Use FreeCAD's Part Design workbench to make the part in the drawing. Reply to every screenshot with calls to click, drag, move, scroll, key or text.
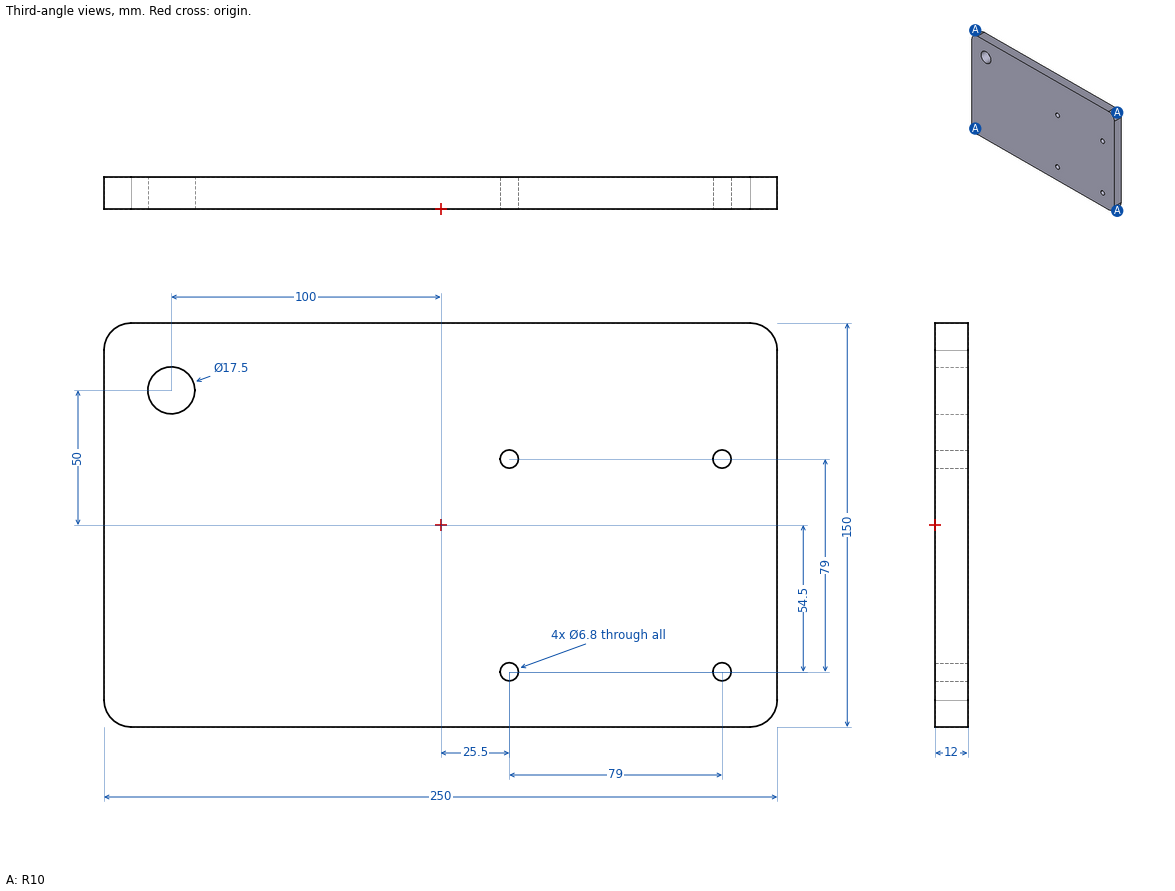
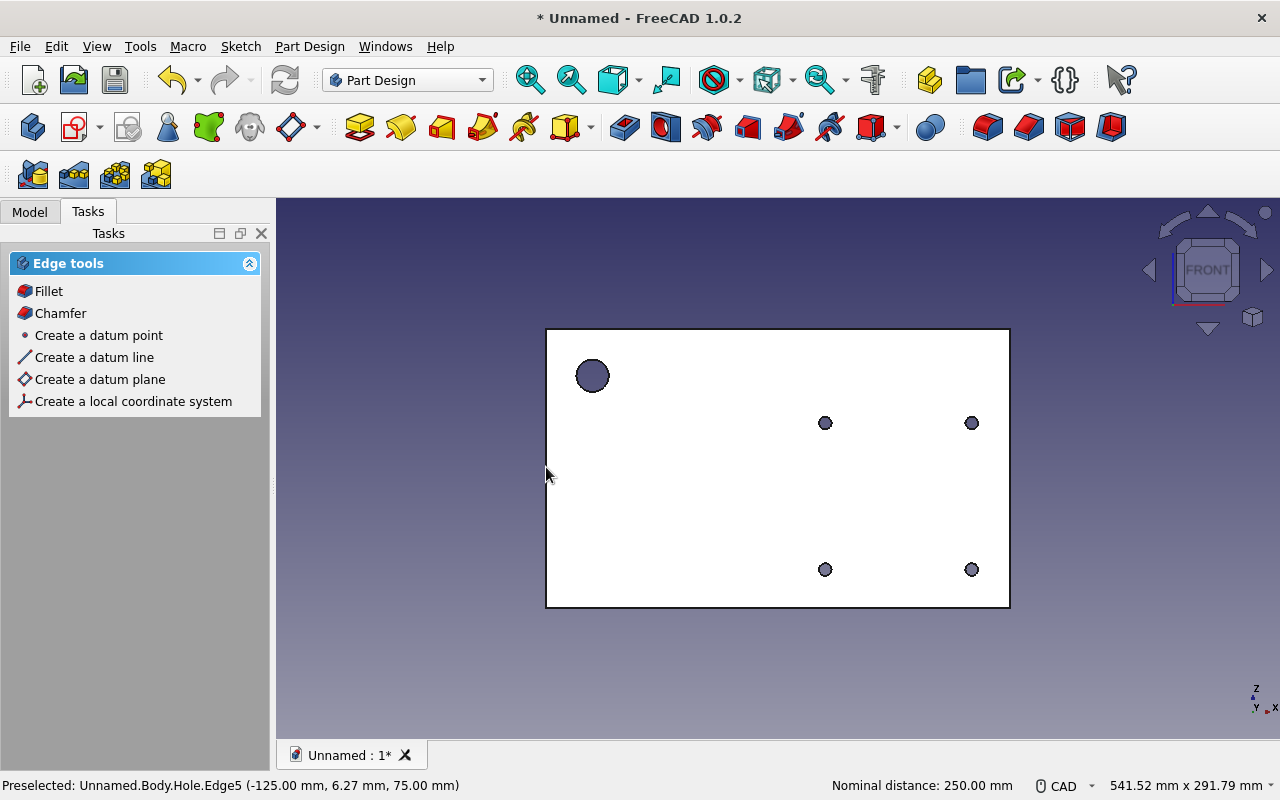
key(3)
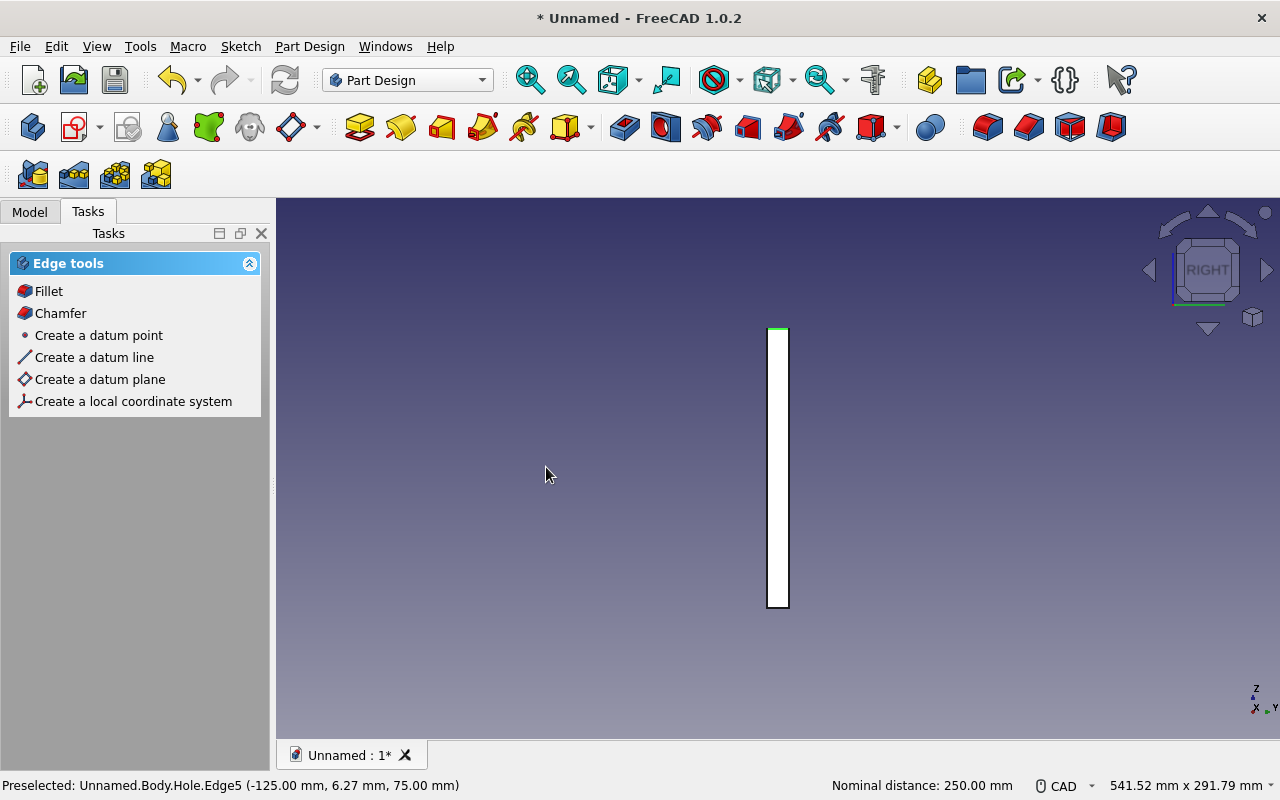
click(778, 607, ctrl)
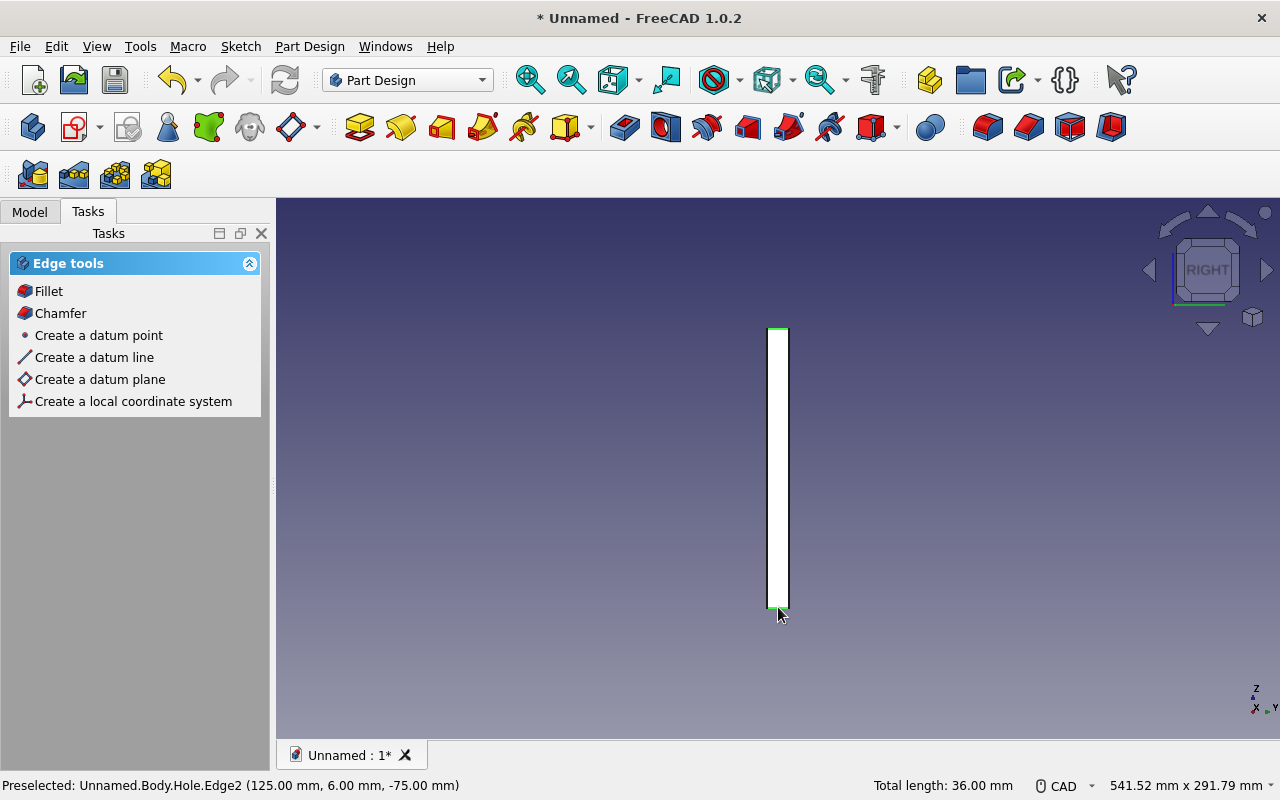
key(5)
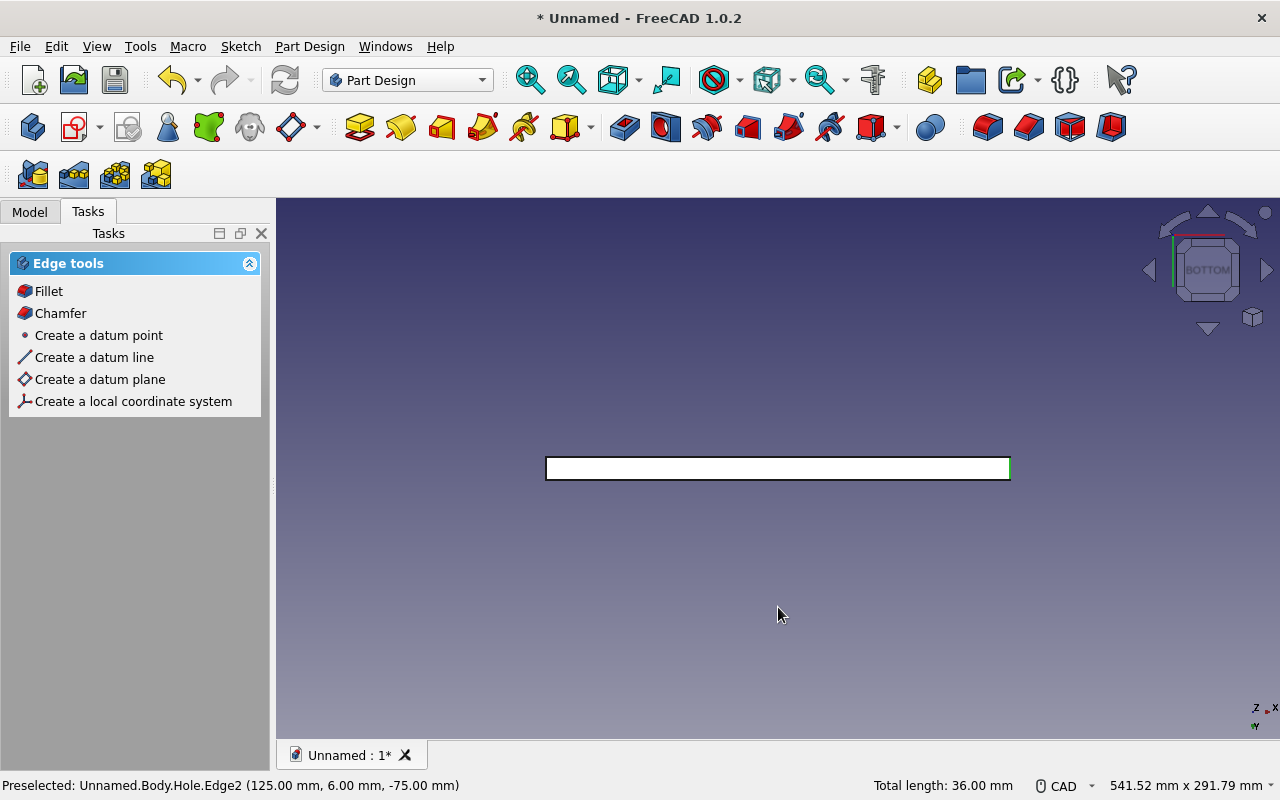
click(546, 468, ctrl)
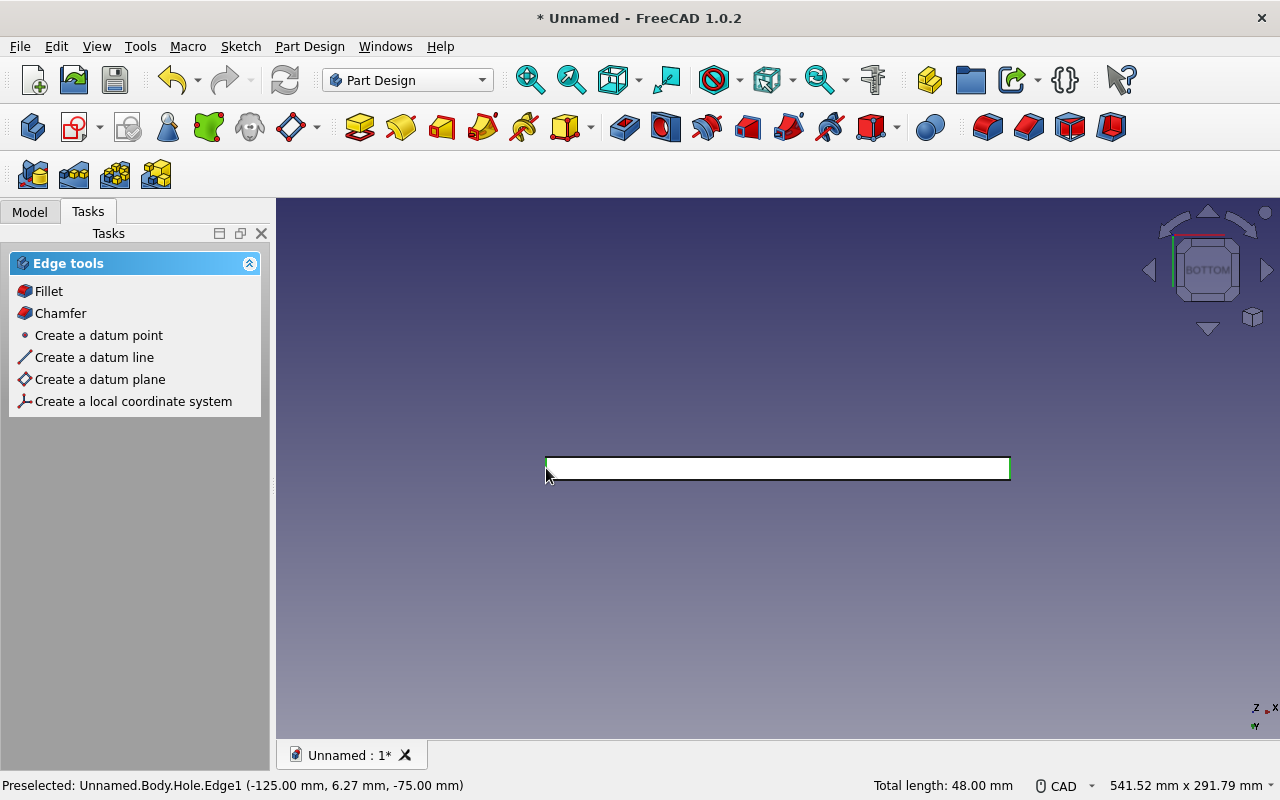
click(988, 128)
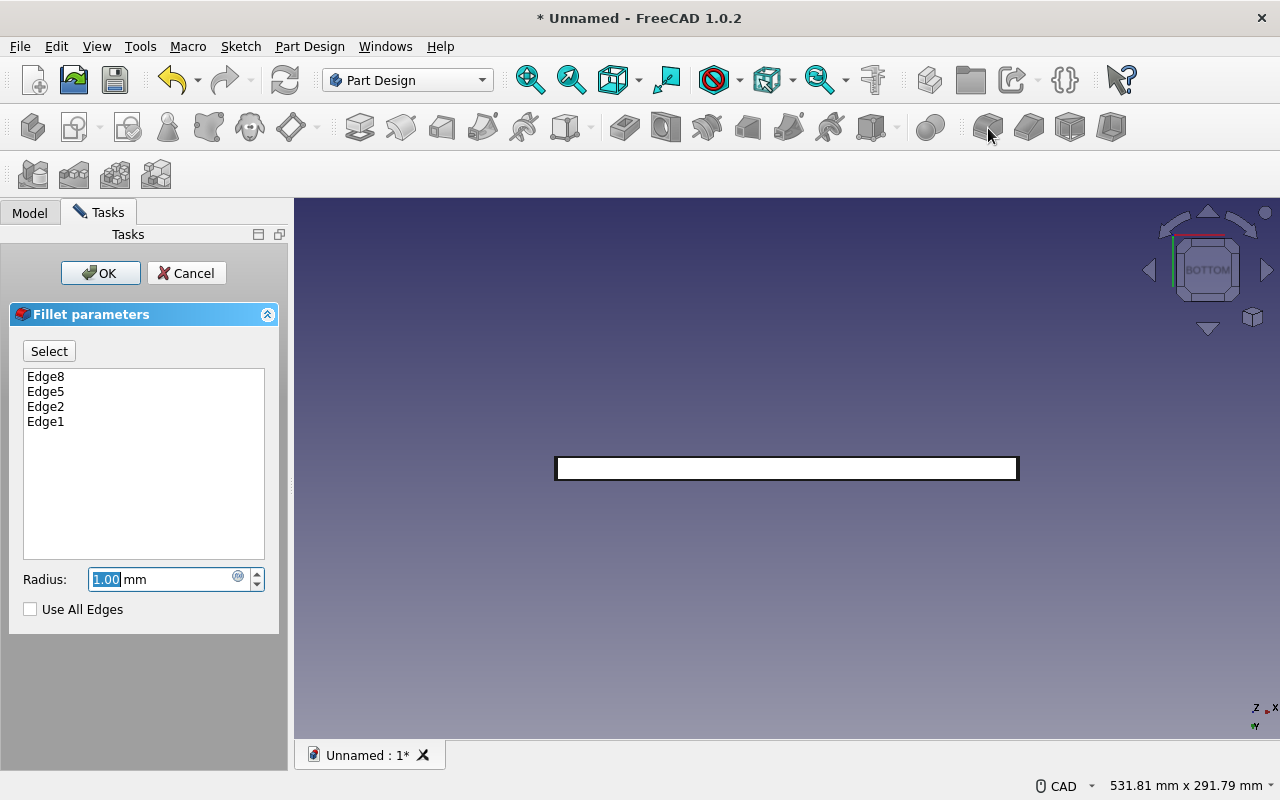
text(10)
key(Tab)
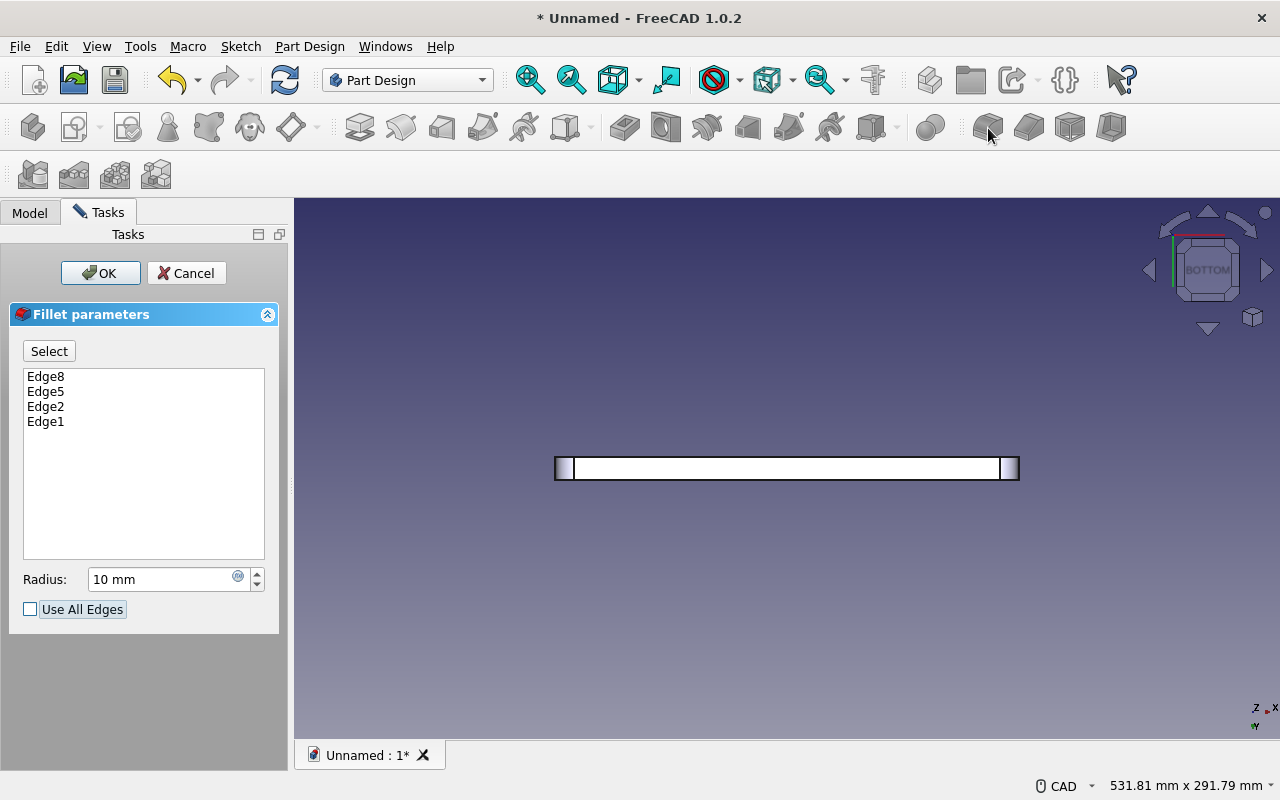
click(101, 273)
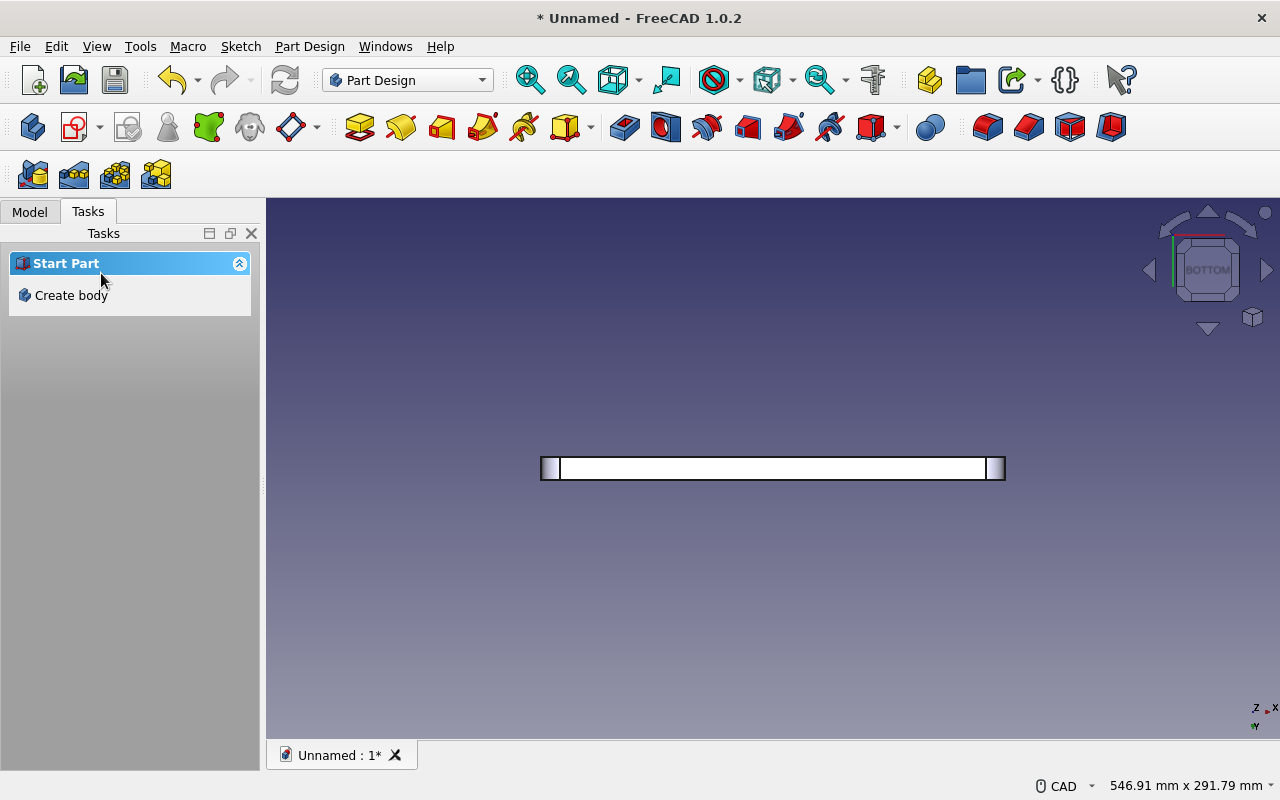
key(0)